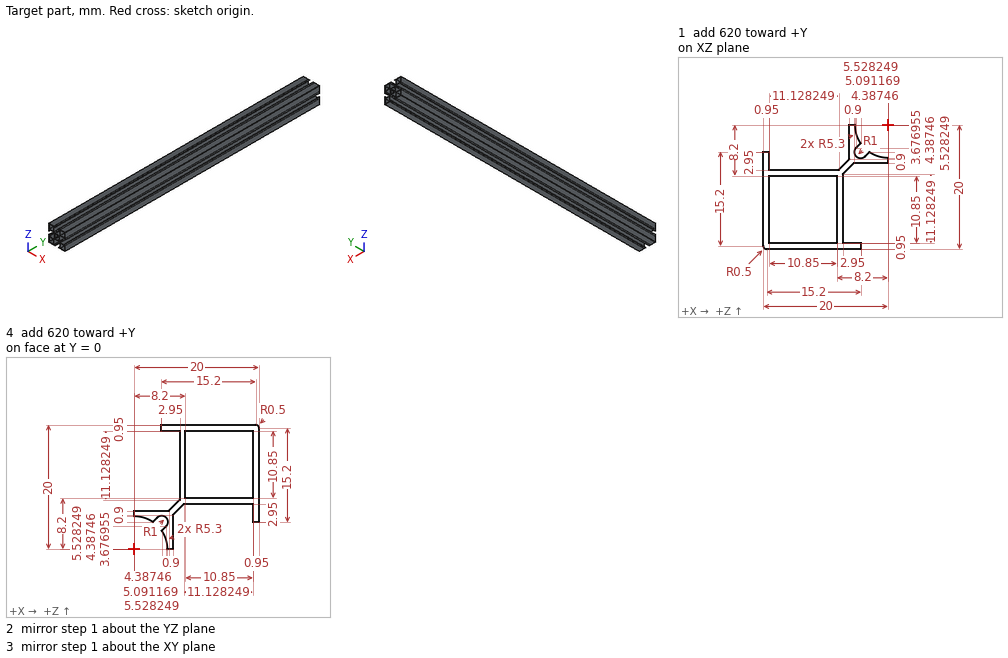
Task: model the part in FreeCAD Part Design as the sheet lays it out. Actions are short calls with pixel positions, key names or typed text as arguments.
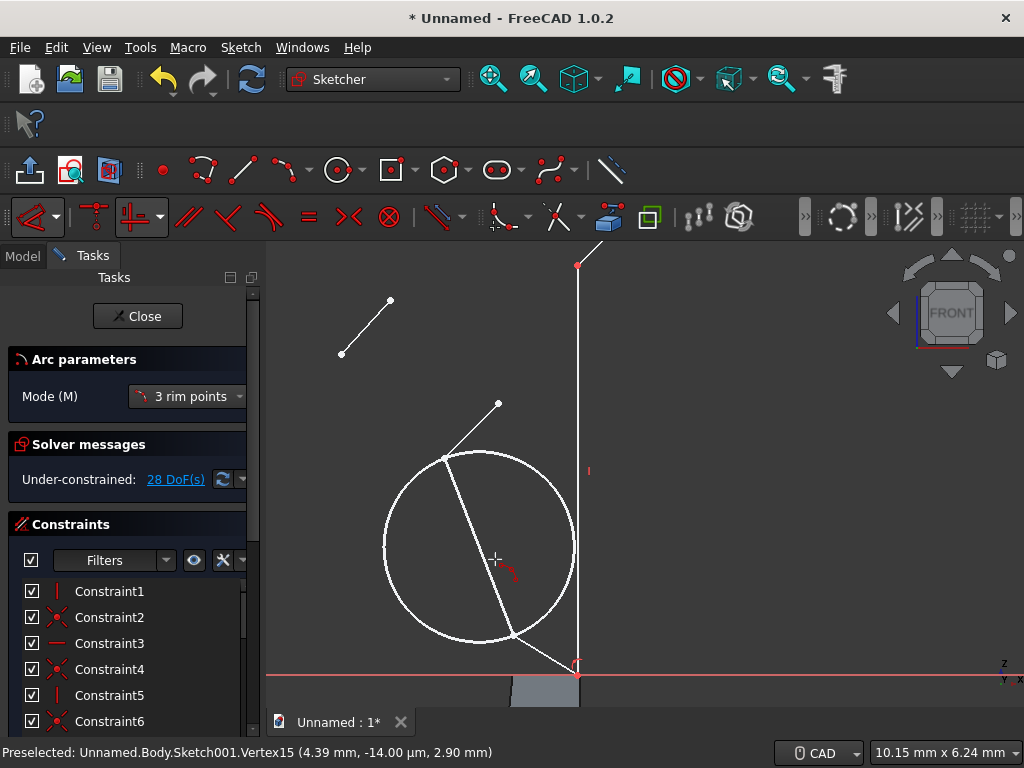
click(495, 559)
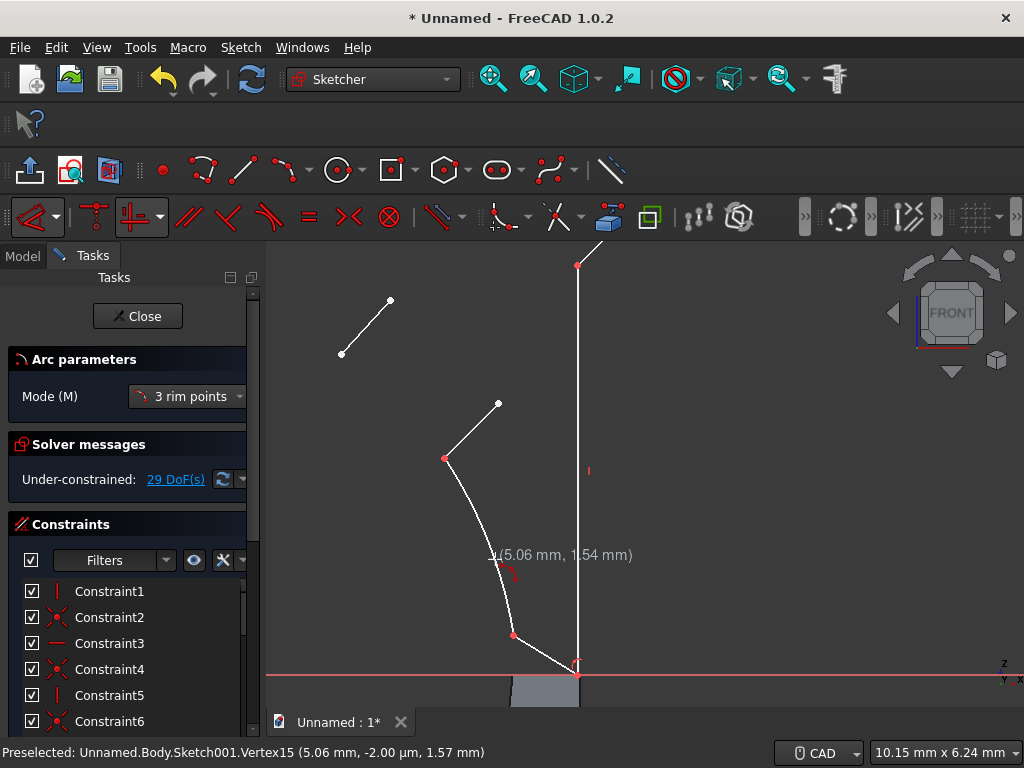
click(499, 404)
click(390, 300)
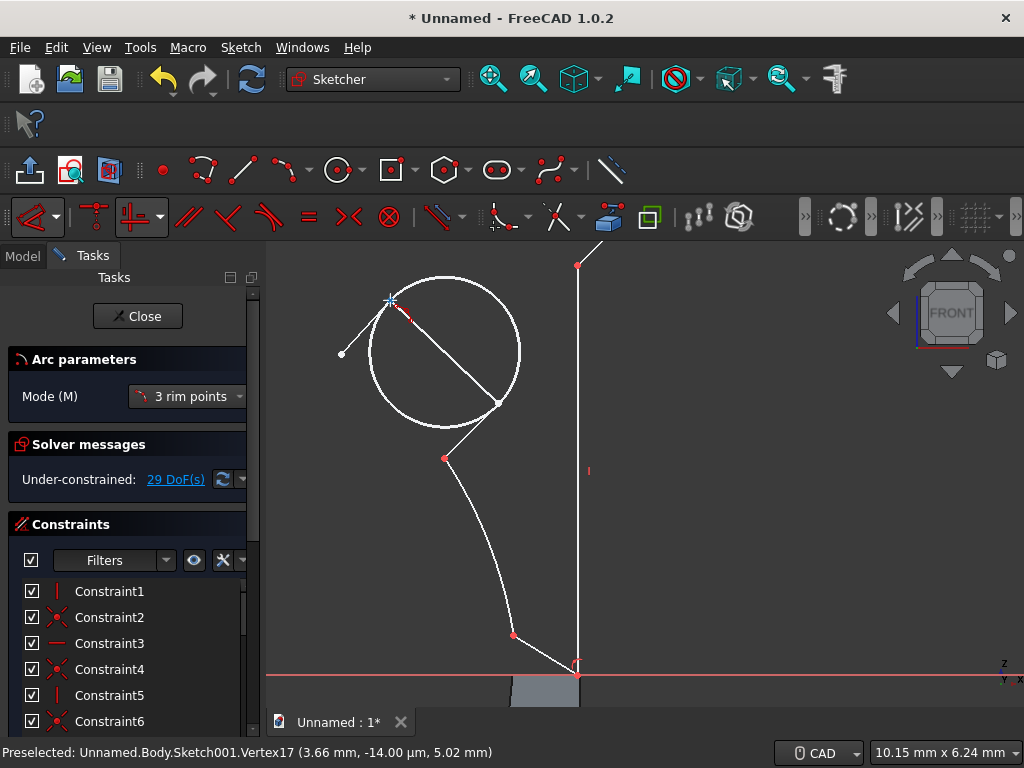
scroll(504, 612, down, 8)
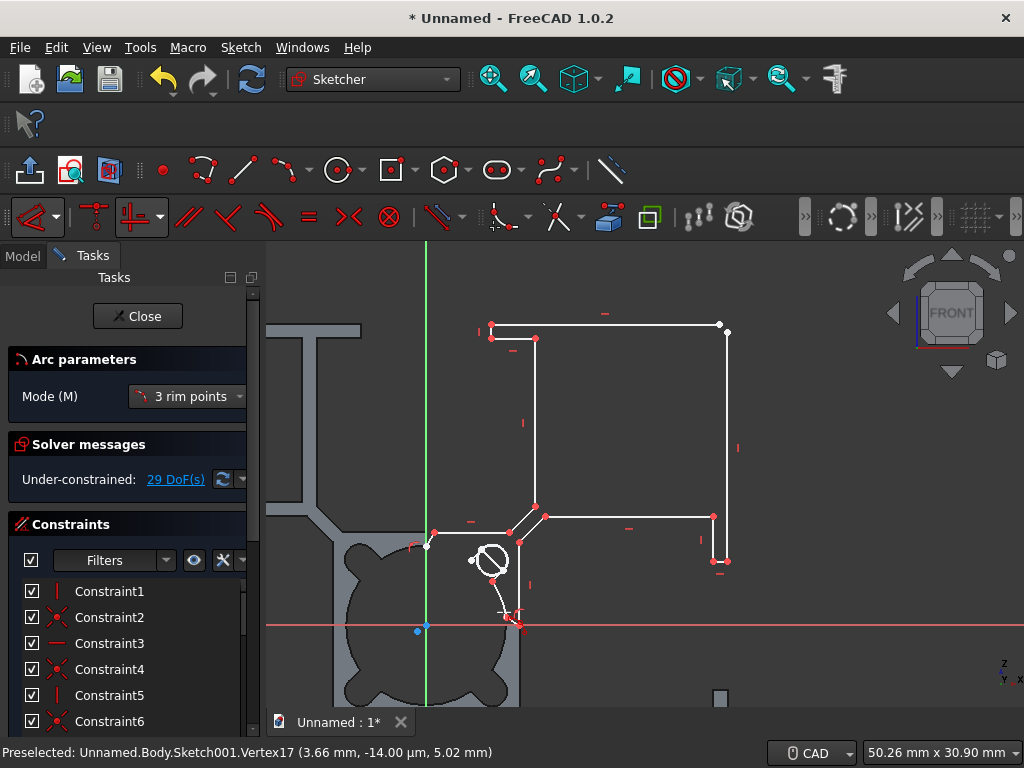
click(503, 549)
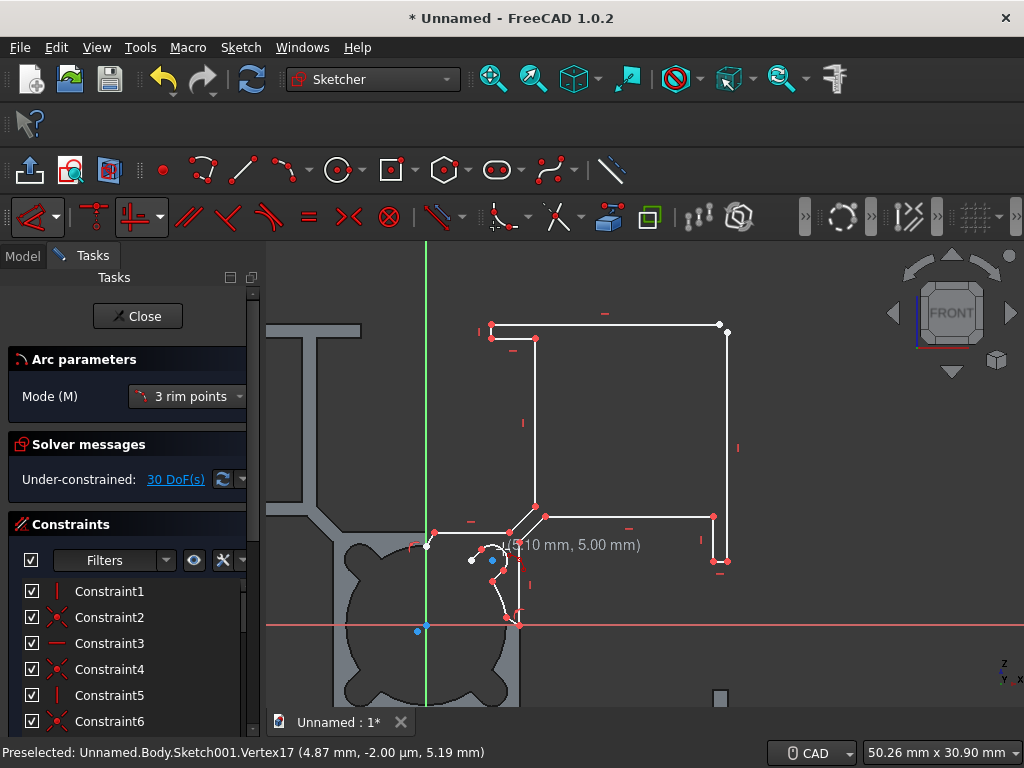
scroll(471, 559, up, 4)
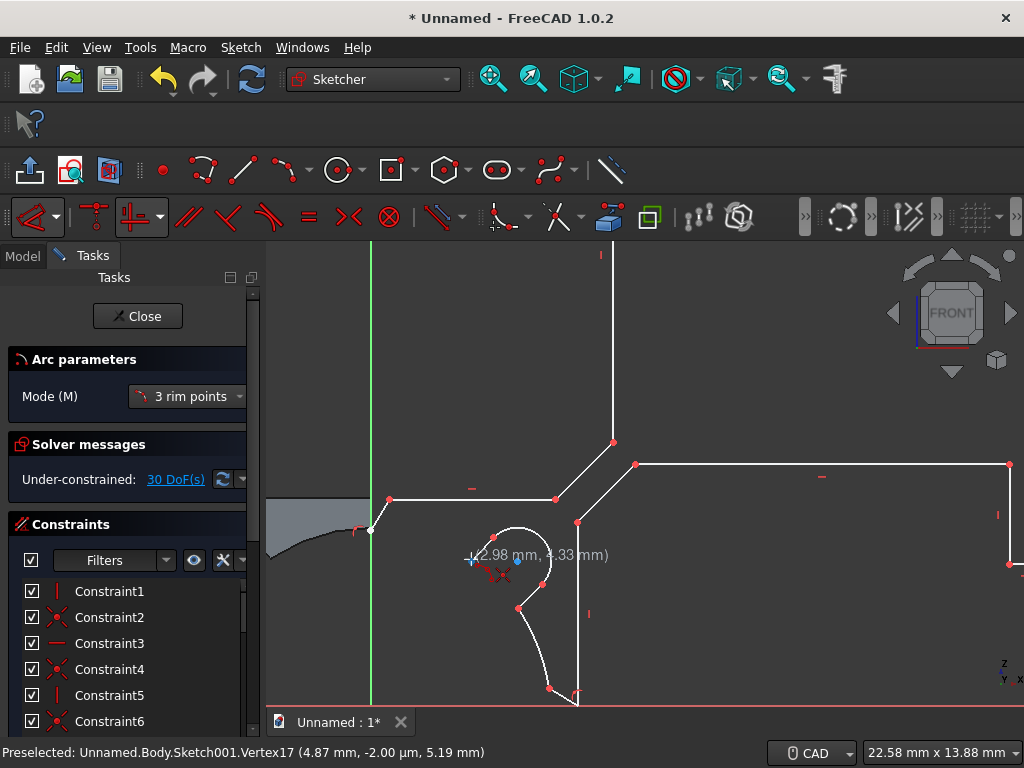
click(471, 562)
click(371, 531)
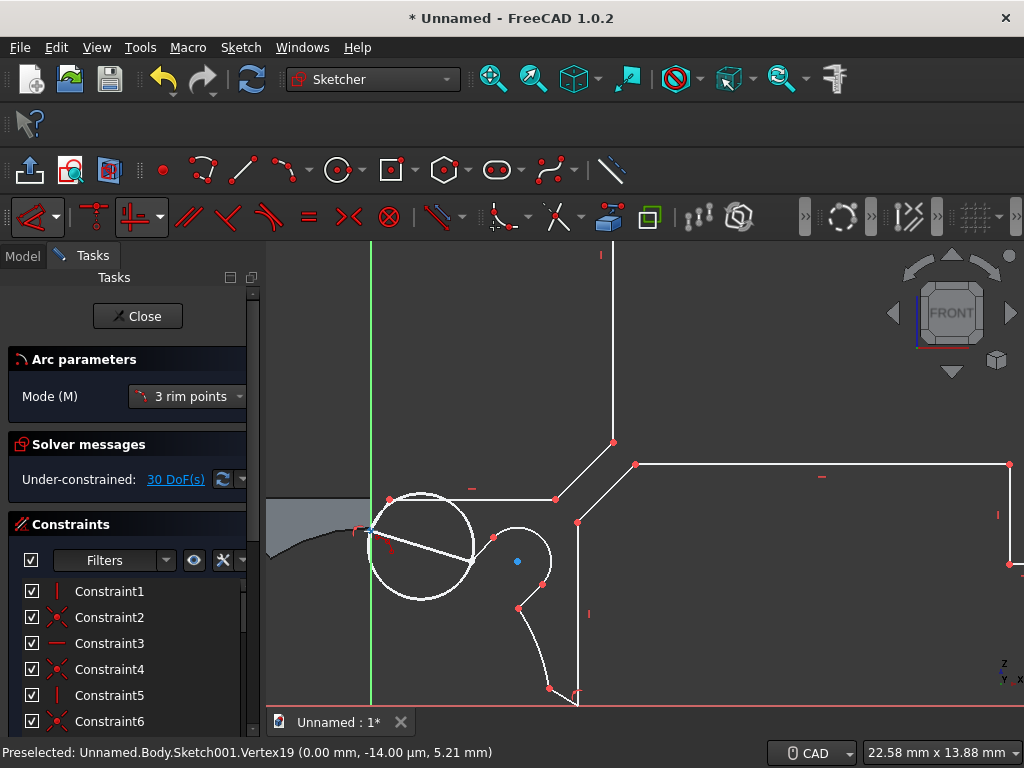
scroll(423, 536, up, 4)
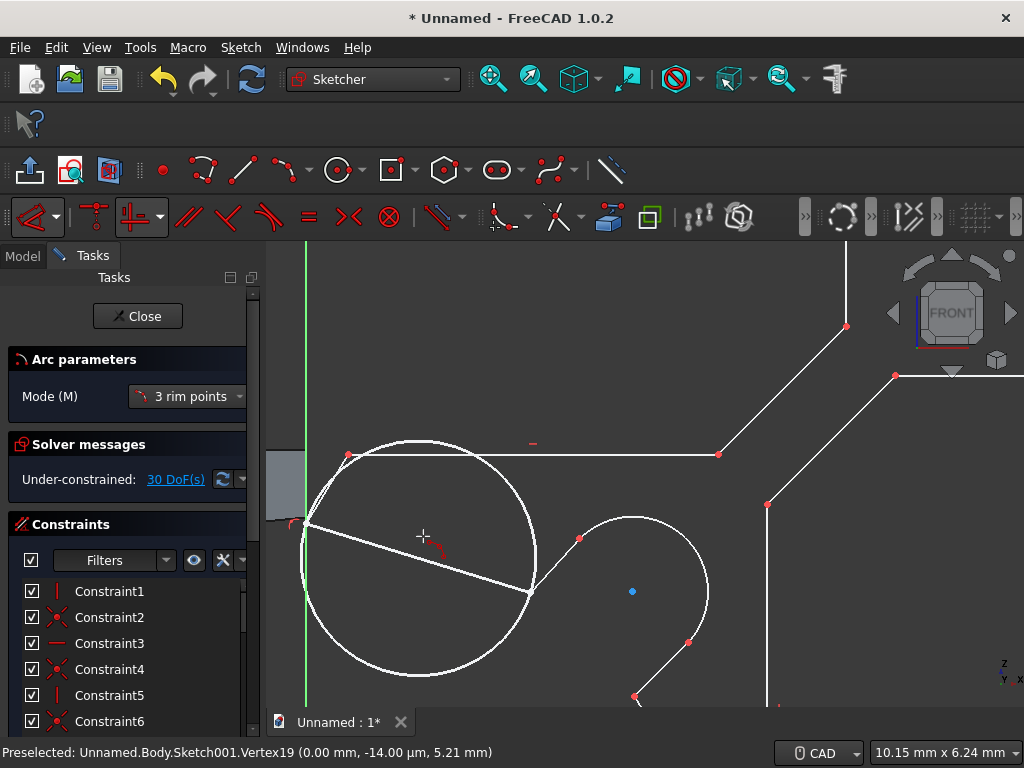
click(422, 535)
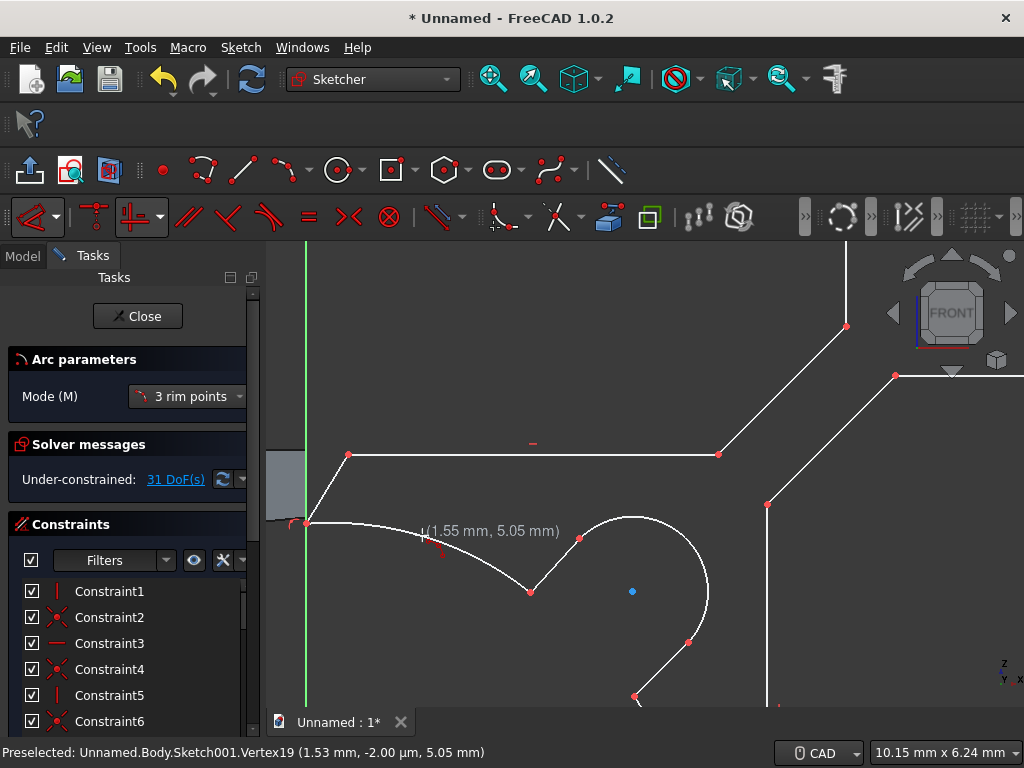
scroll(456, 552, down, 8)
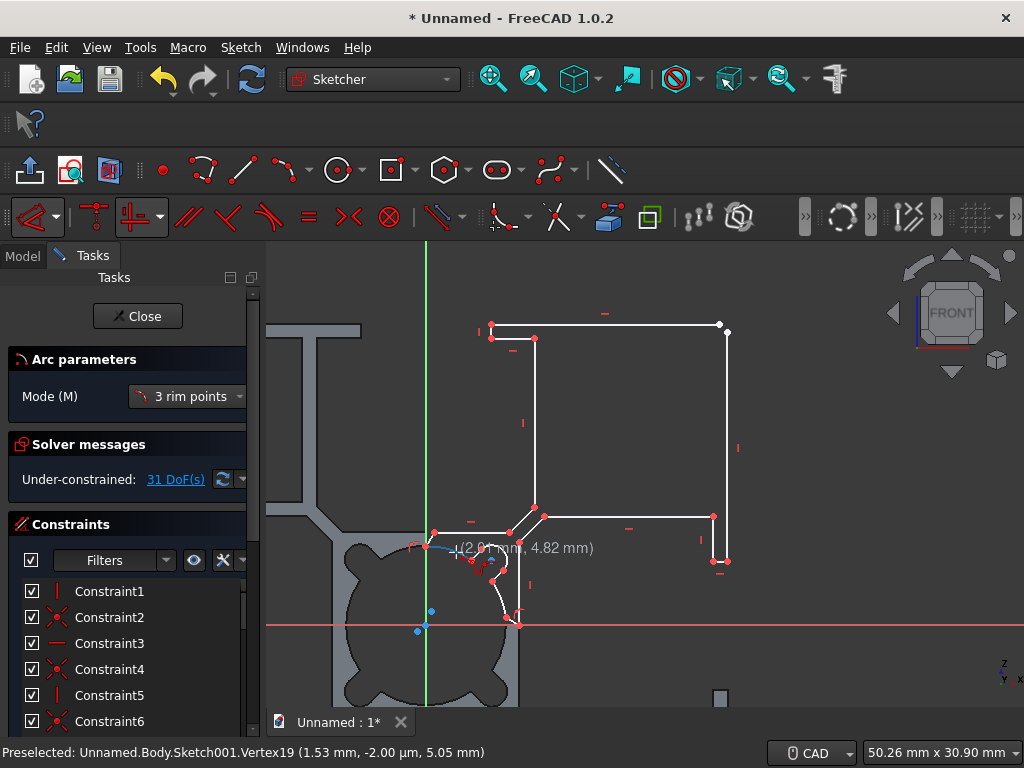
scroll(720, 324, up, 2)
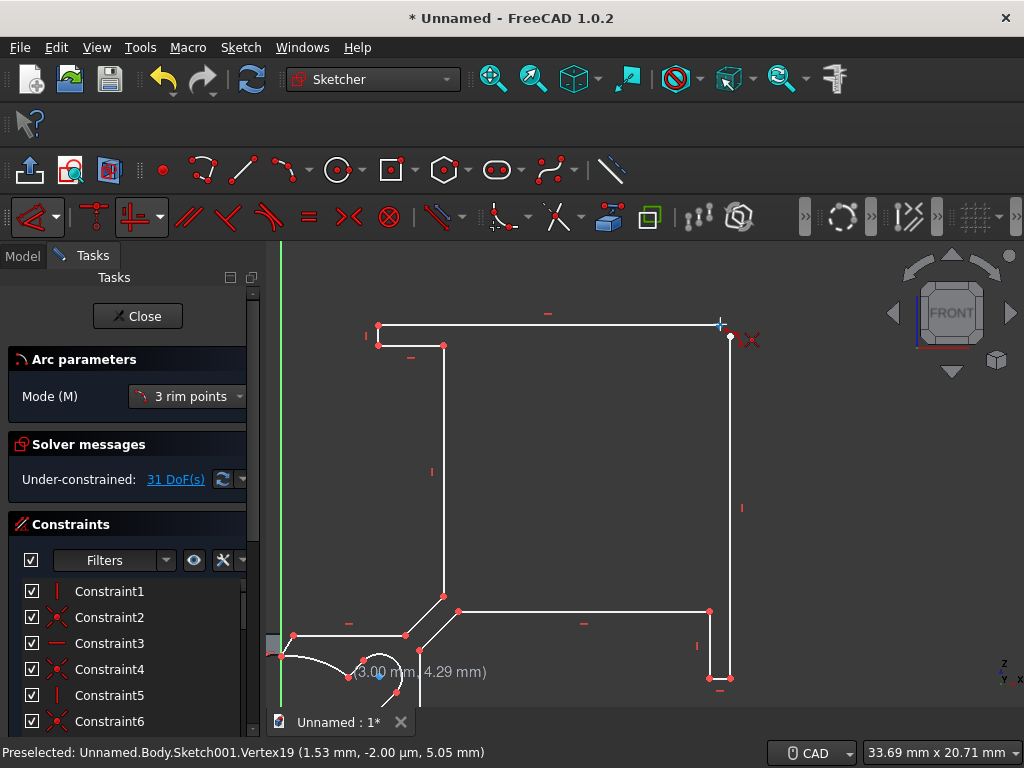
click(719, 325)
click(730, 337)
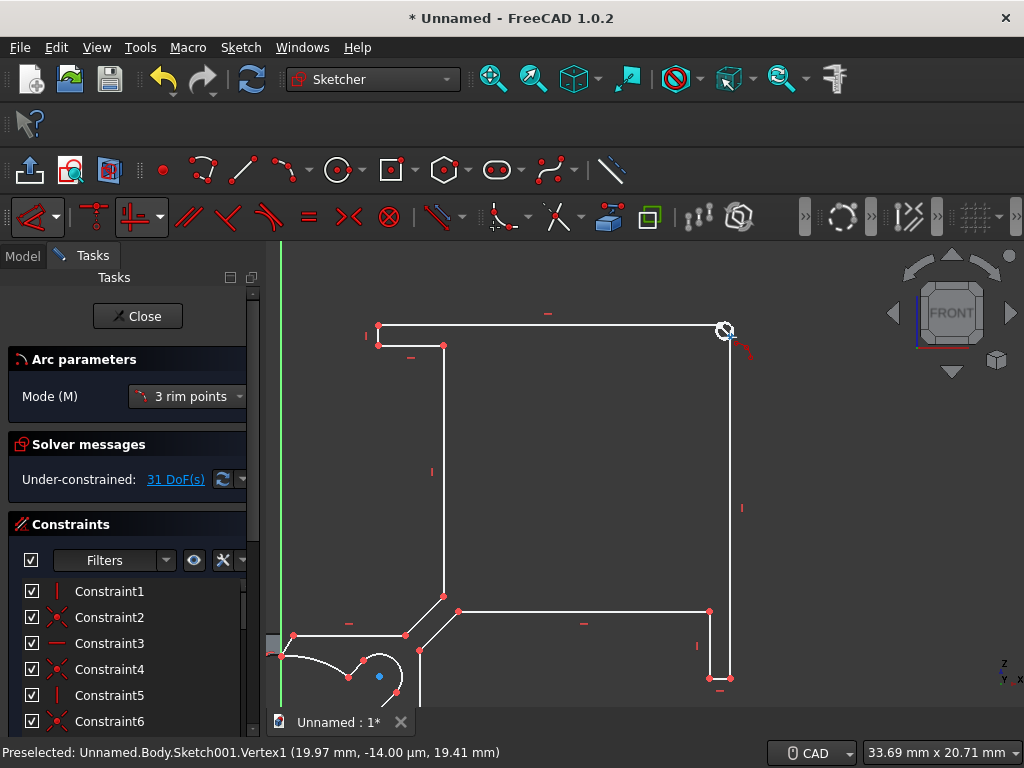
scroll(728, 327, up, 8)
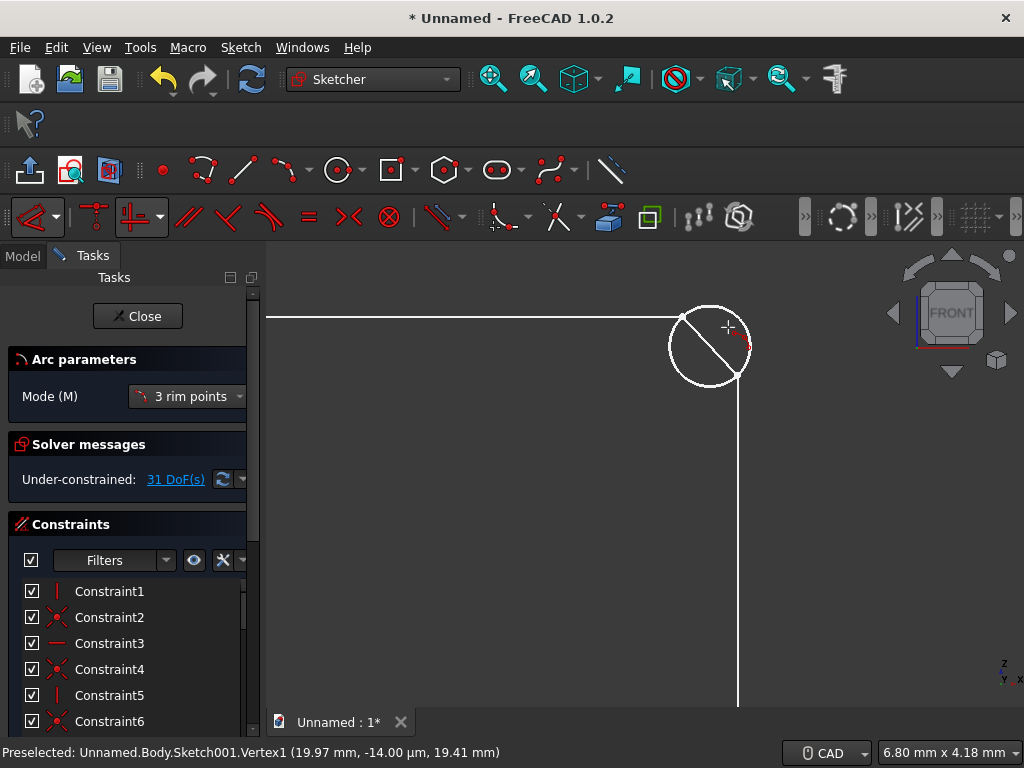
click(724, 326)